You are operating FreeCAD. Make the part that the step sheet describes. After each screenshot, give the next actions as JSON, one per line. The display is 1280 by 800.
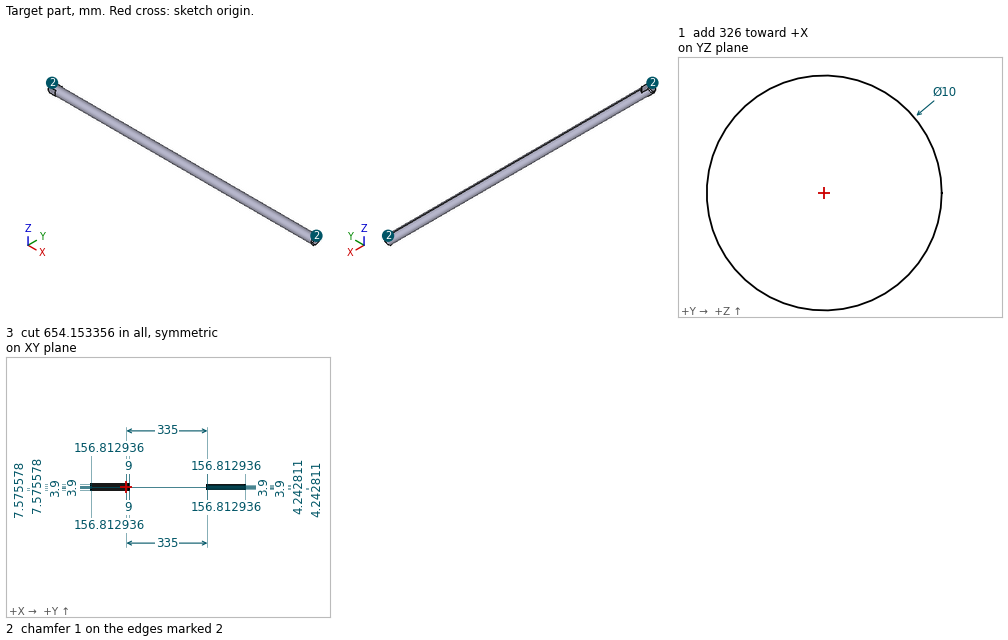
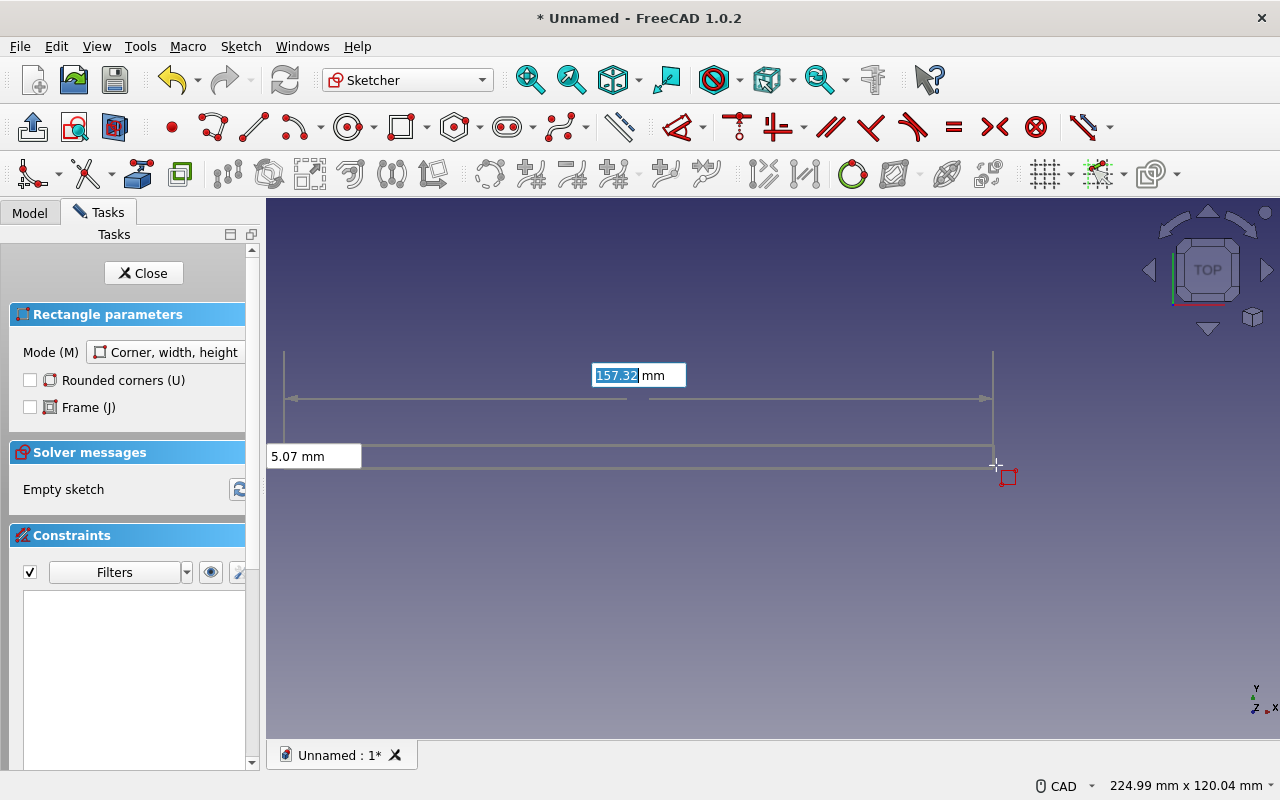
{"action": "left_click", "coordinate": [991, 463]}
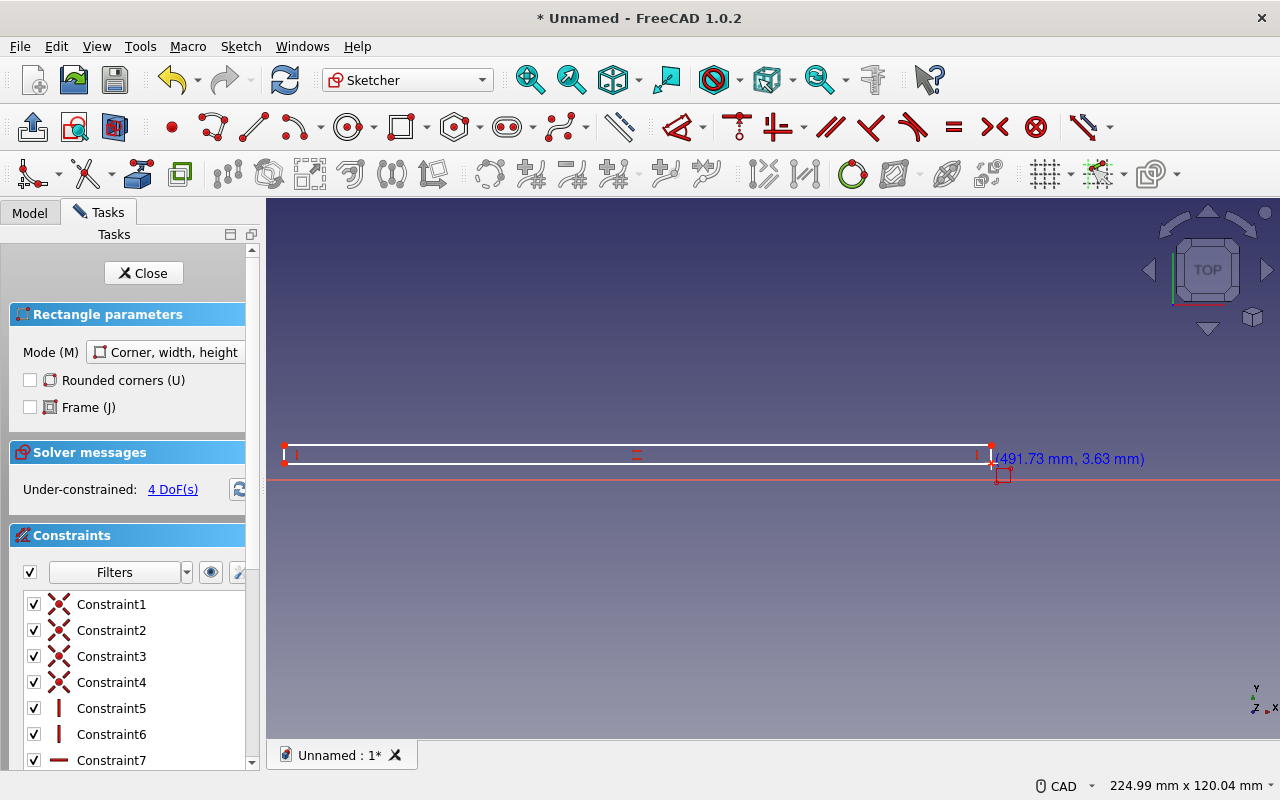
{"action": "scroll", "coordinate": [997, 465], "scroll_direction": "down", "scroll_amount": 8}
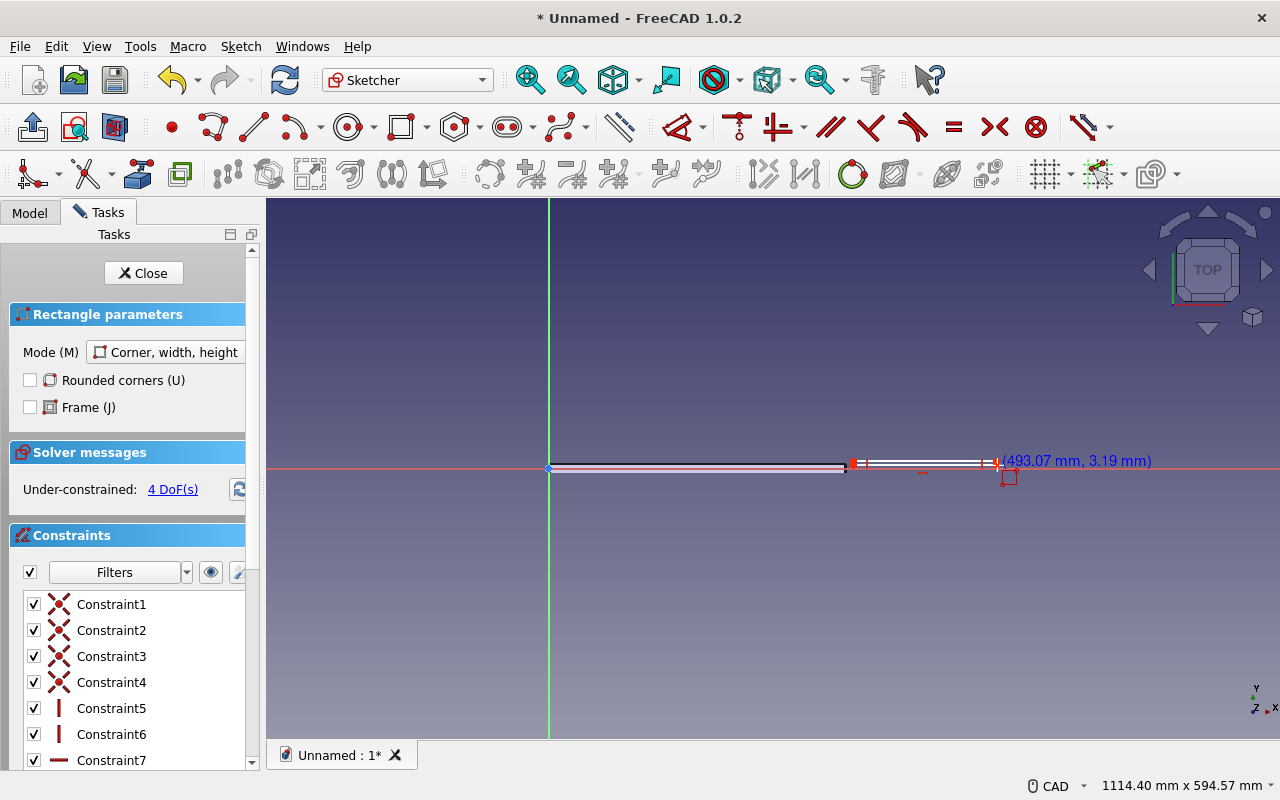
{"action": "scroll", "coordinate": [854, 472], "scroll_direction": "up", "scroll_amount": 8}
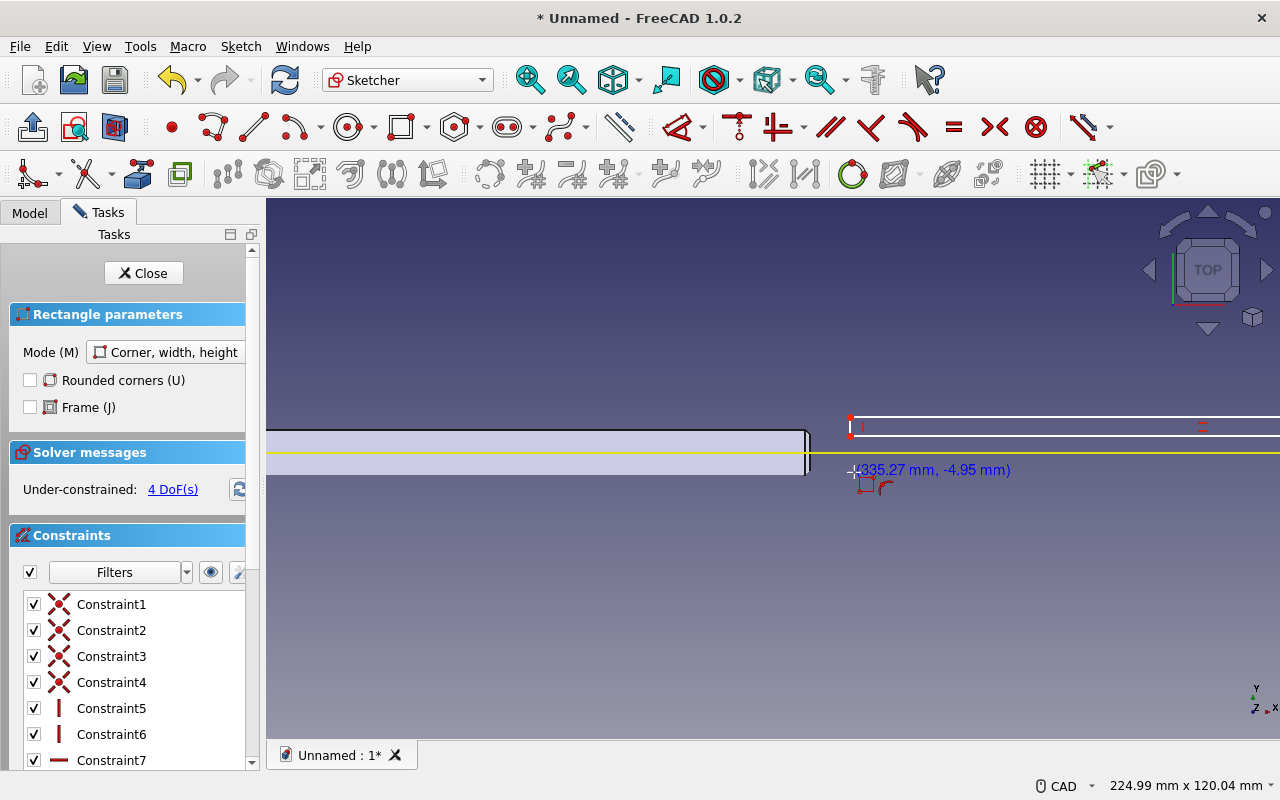
{"action": "left_click", "coordinate": [850, 470]}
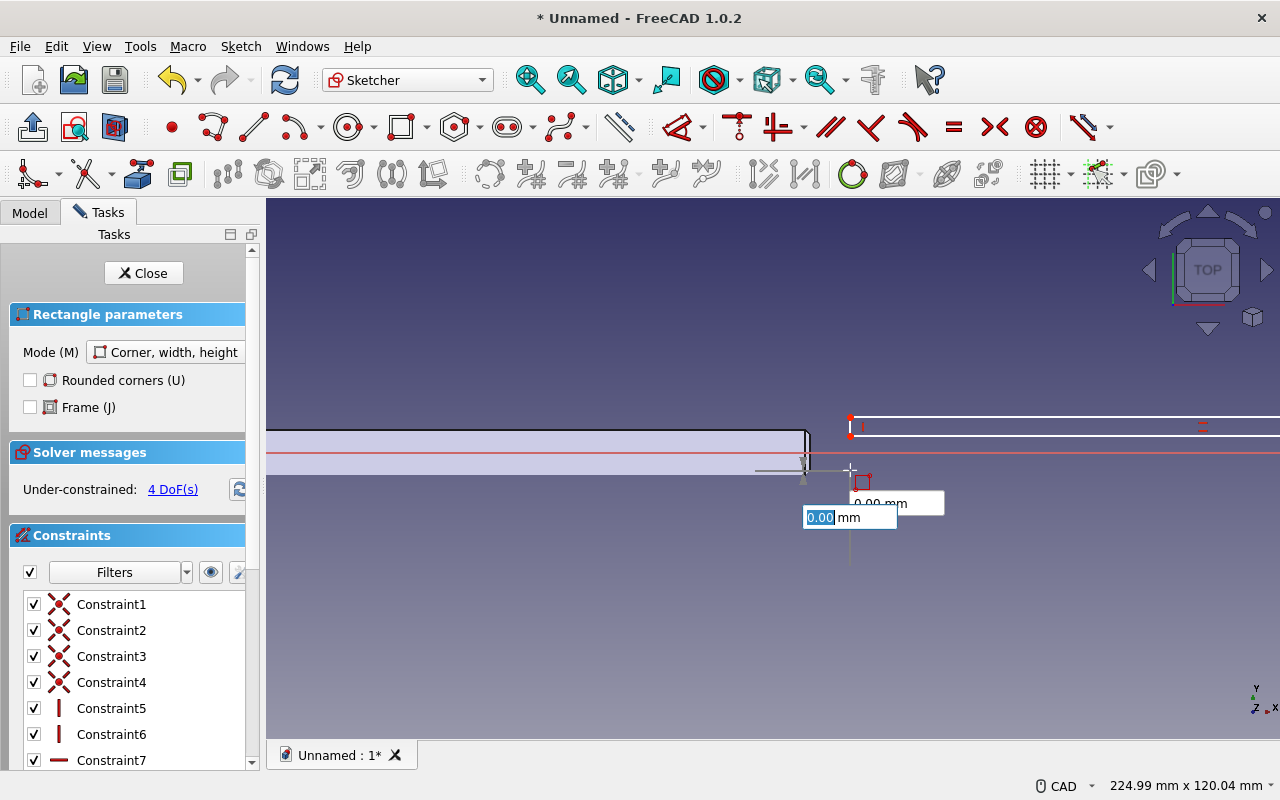
{"action": "scroll", "coordinate": [853, 473], "scroll_direction": "down", "scroll_amount": 8}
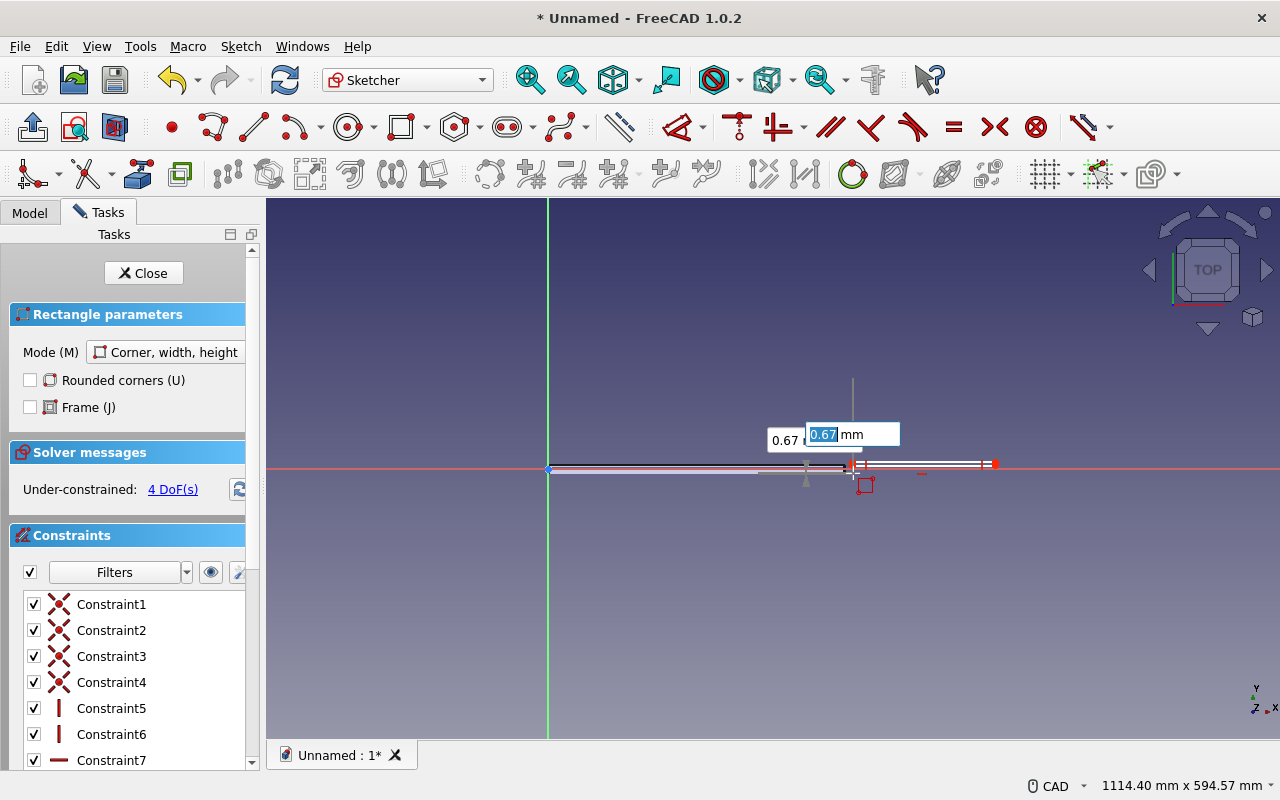
{"action": "scroll", "coordinate": [996, 477], "scroll_direction": "up", "scroll_amount": 4}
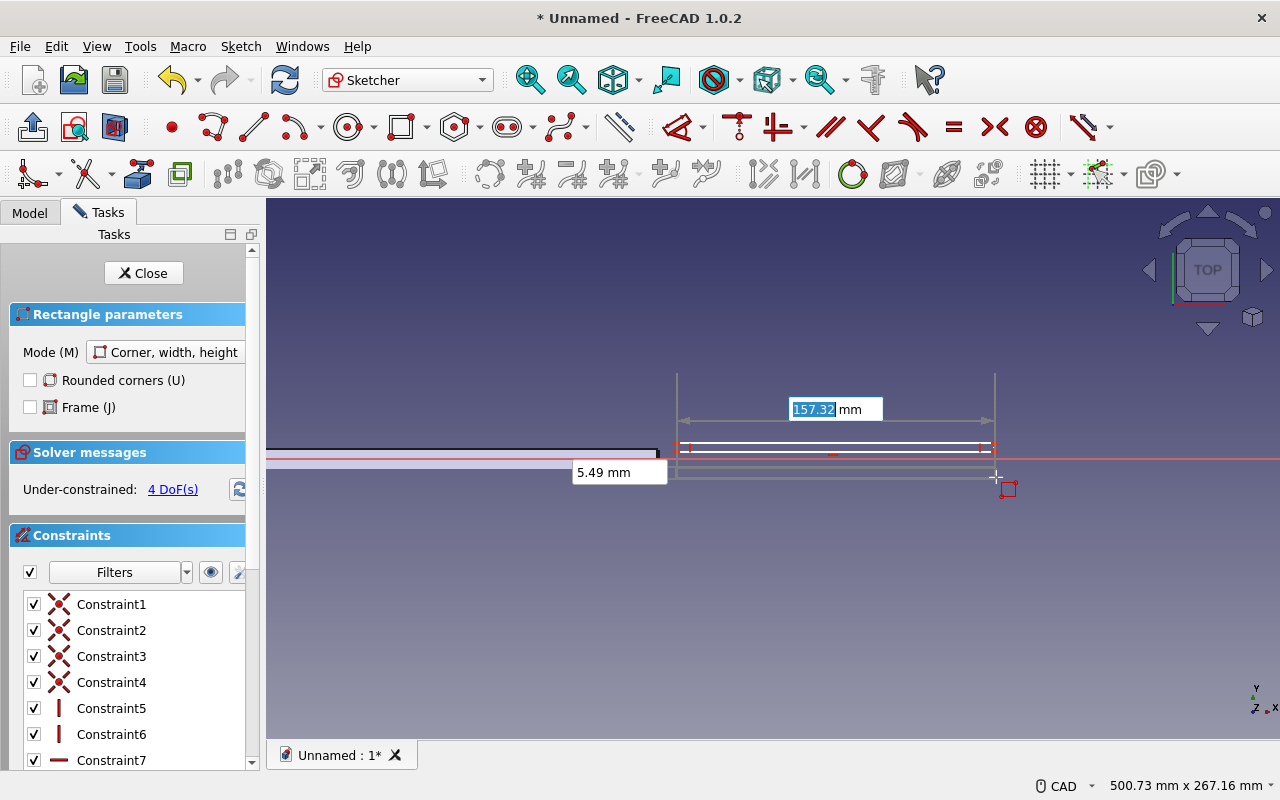
{"action": "left_click", "coordinate": [994, 476]}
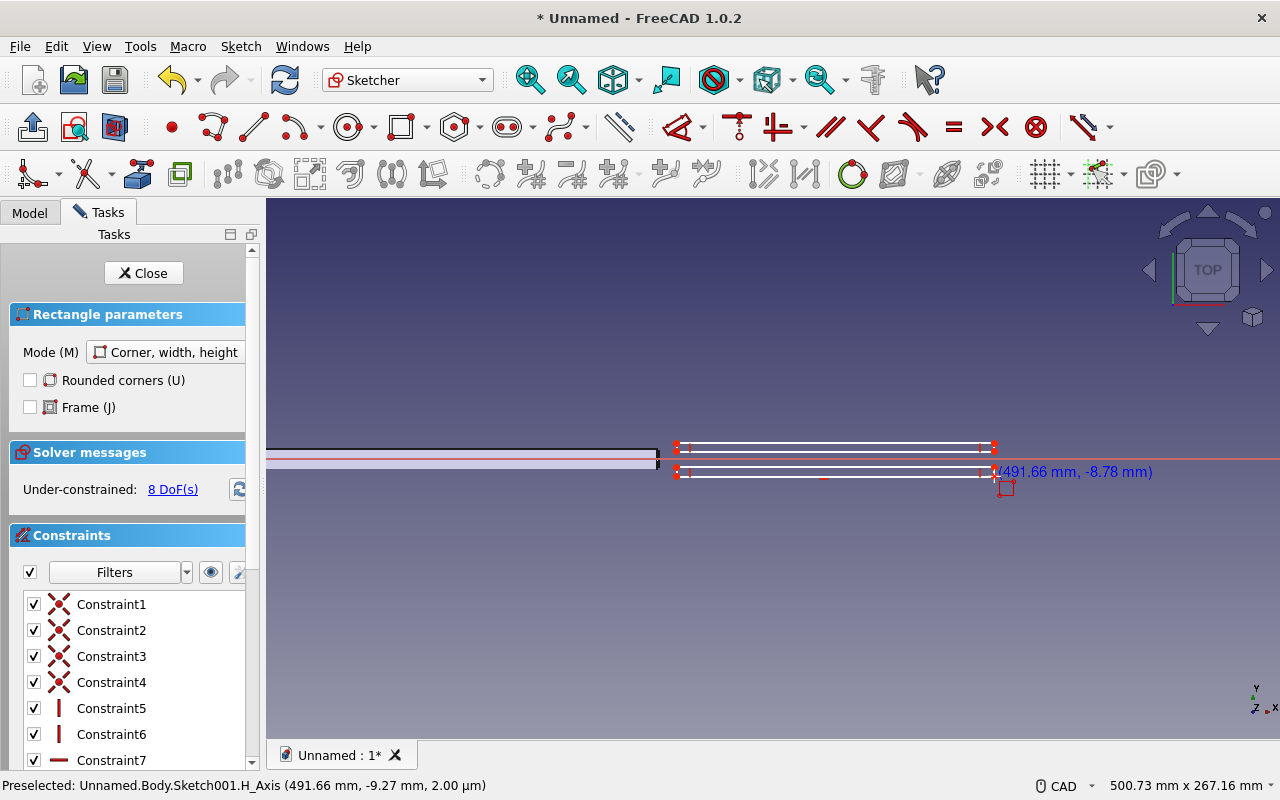
{"action": "scroll", "coordinate": [996, 476], "scroll_direction": "down", "scroll_amount": 4}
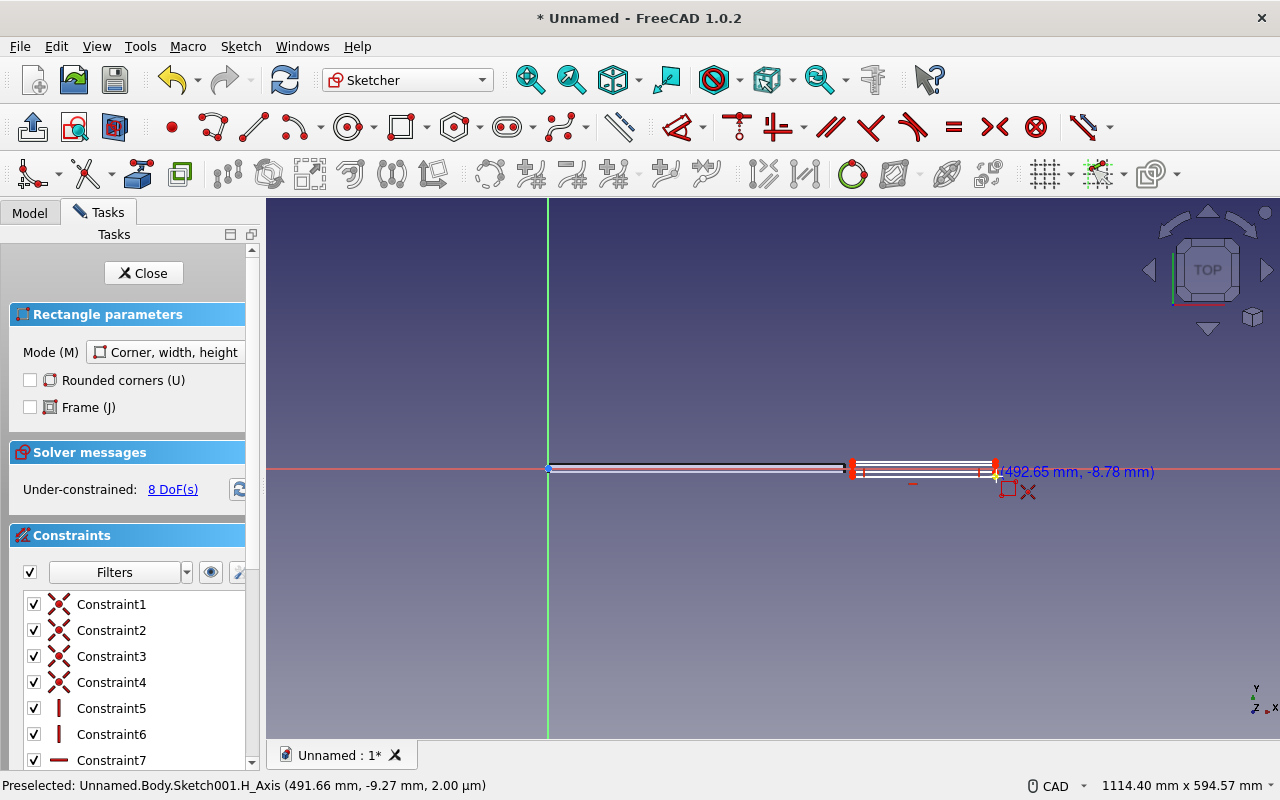
{"action": "scroll", "coordinate": [414, 458], "scroll_direction": "up", "scroll_amount": 5}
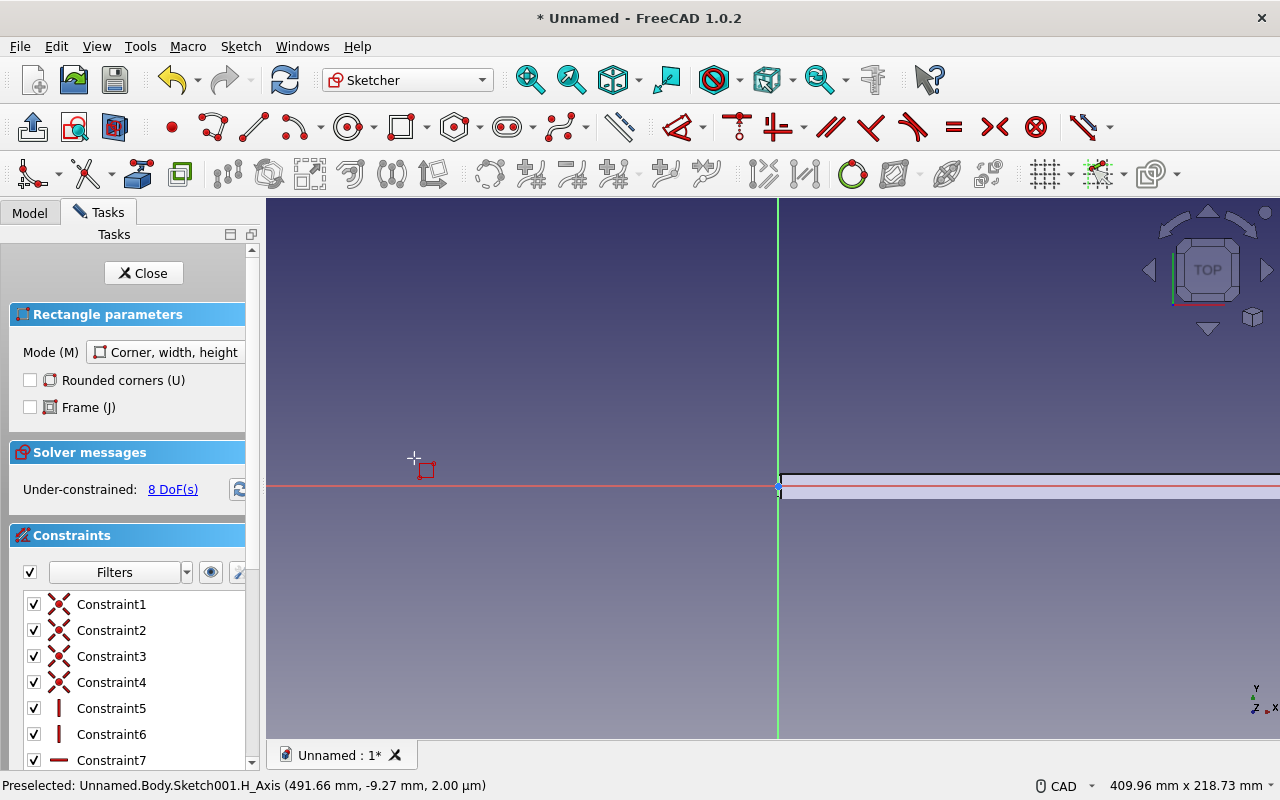
{"action": "left_click", "coordinate": [413, 458]}